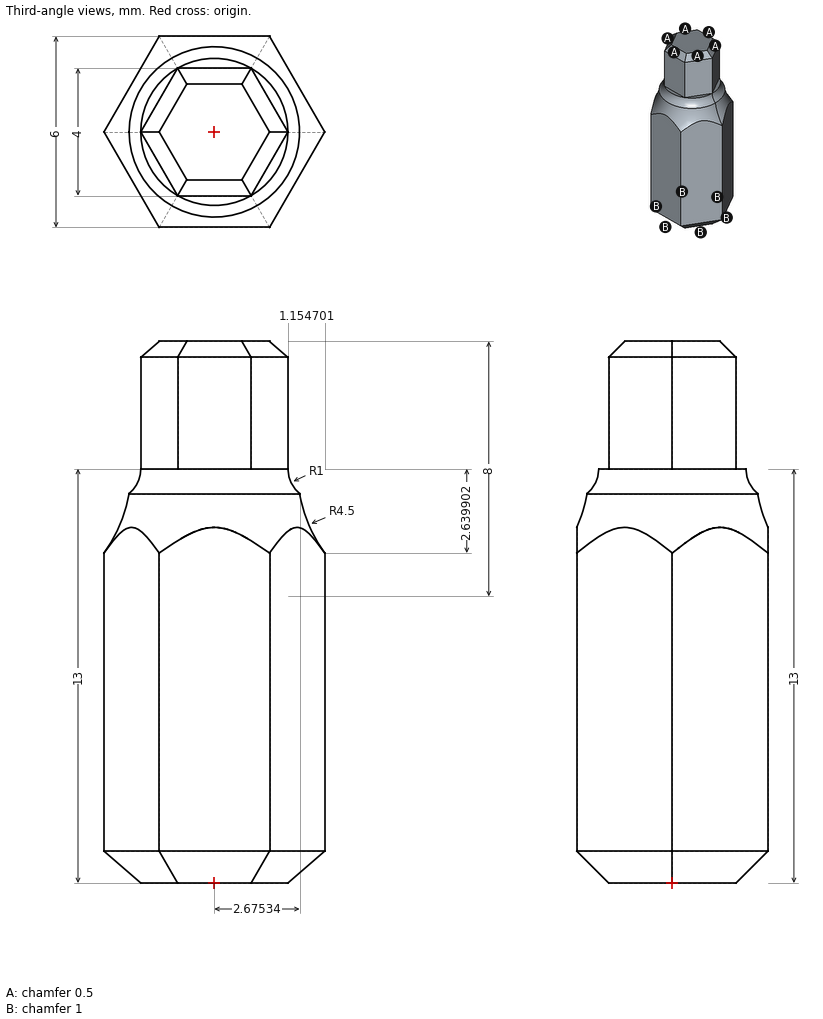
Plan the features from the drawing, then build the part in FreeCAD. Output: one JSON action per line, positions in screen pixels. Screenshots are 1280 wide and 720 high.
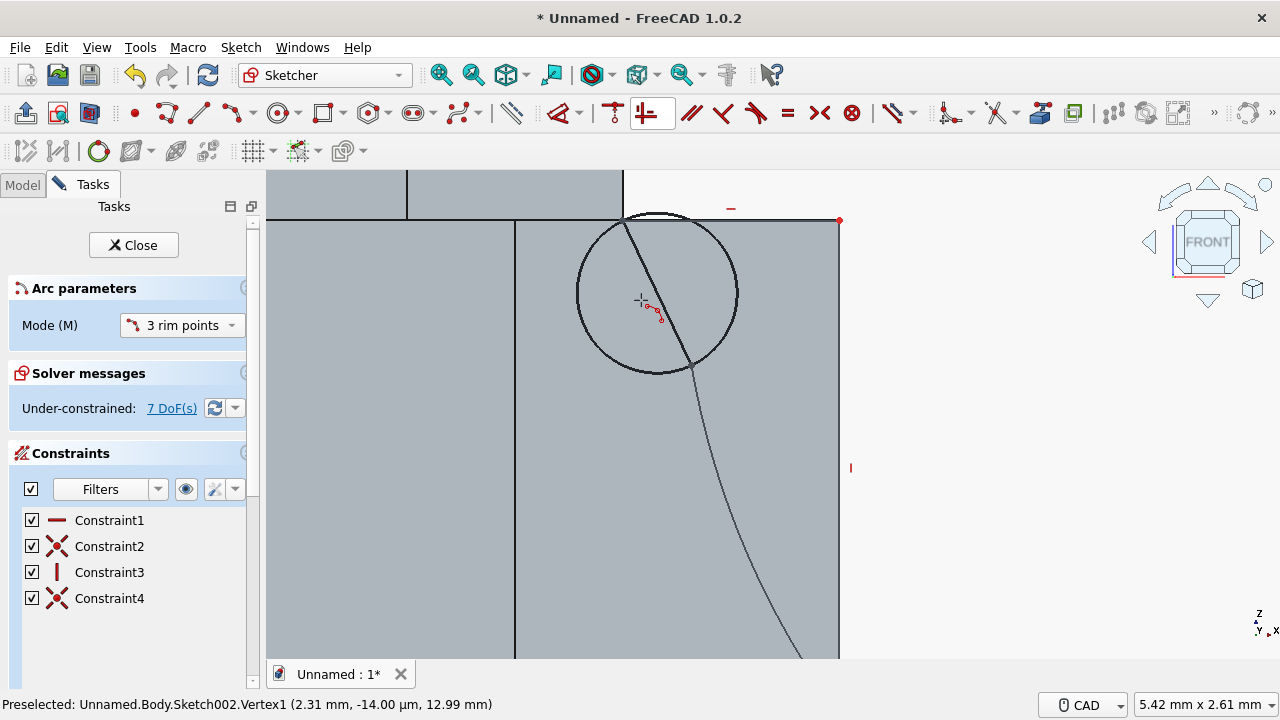
{"action": "left_click", "coordinate": [641, 300]}
{"action": "key", "text": "Escape"}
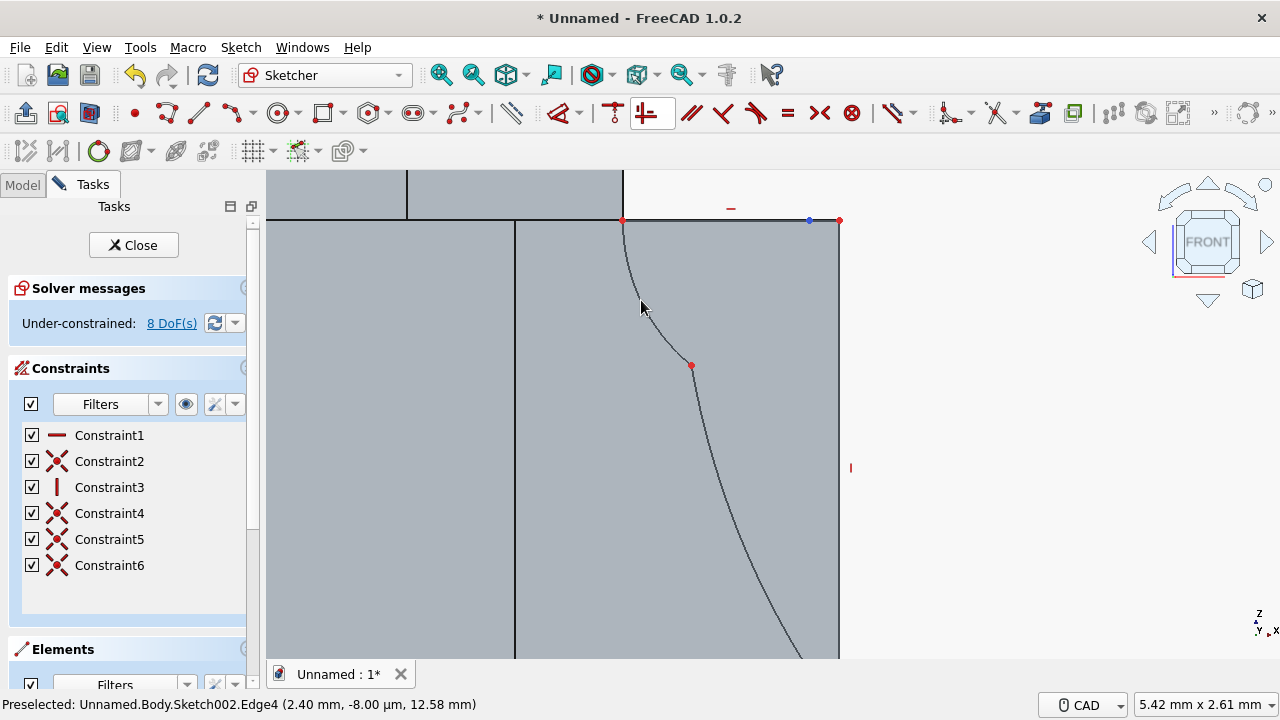
{"action": "left_click", "coordinate": [558, 114]}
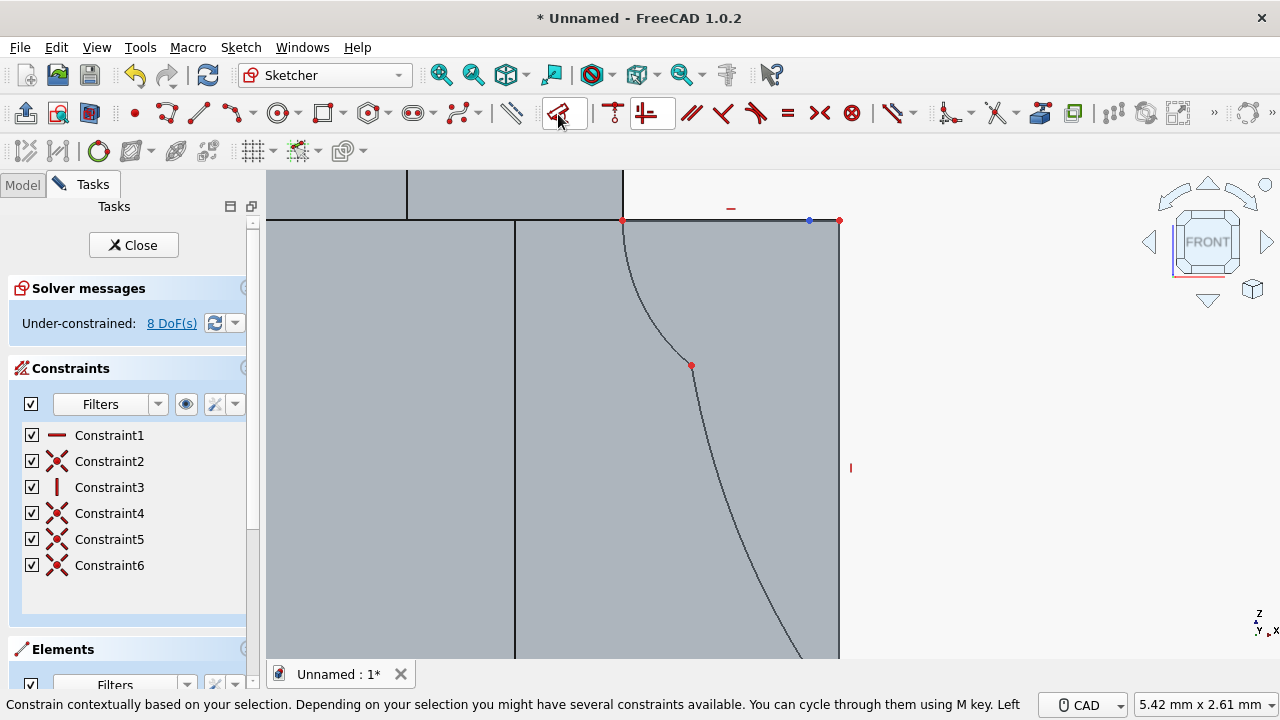
{"action": "left_click", "coordinate": [719, 477]}
{"action": "left_click", "coordinate": [689, 487]}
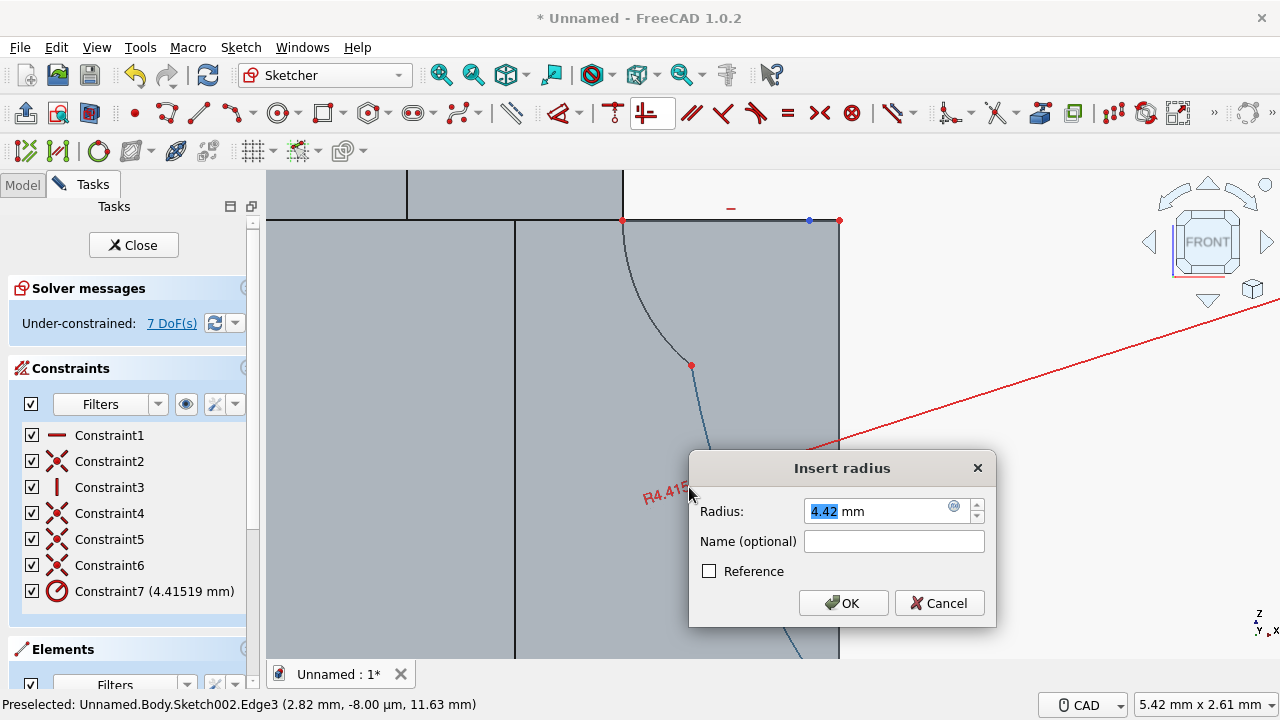
{"action": "type", "text": "4.5"}
{"action": "key", "text": "Return"}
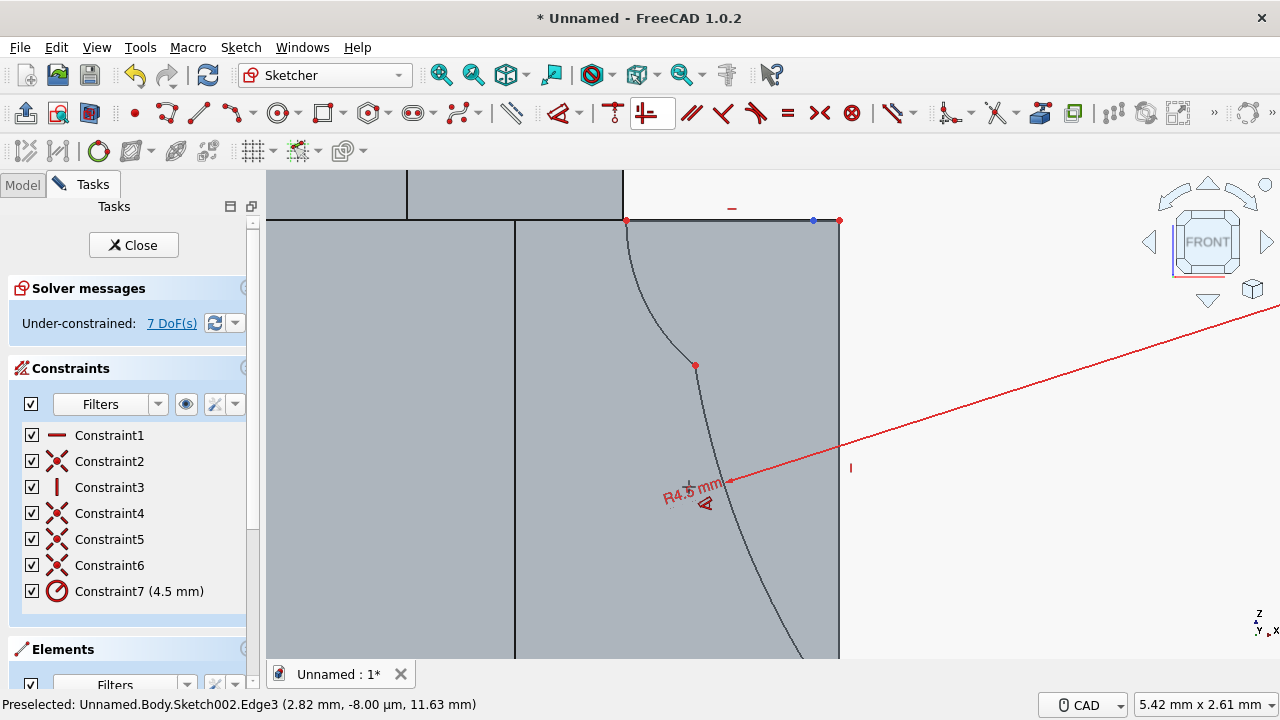
{"action": "left_click", "coordinate": [633, 270]}
{"action": "left_click", "coordinate": [602, 278]}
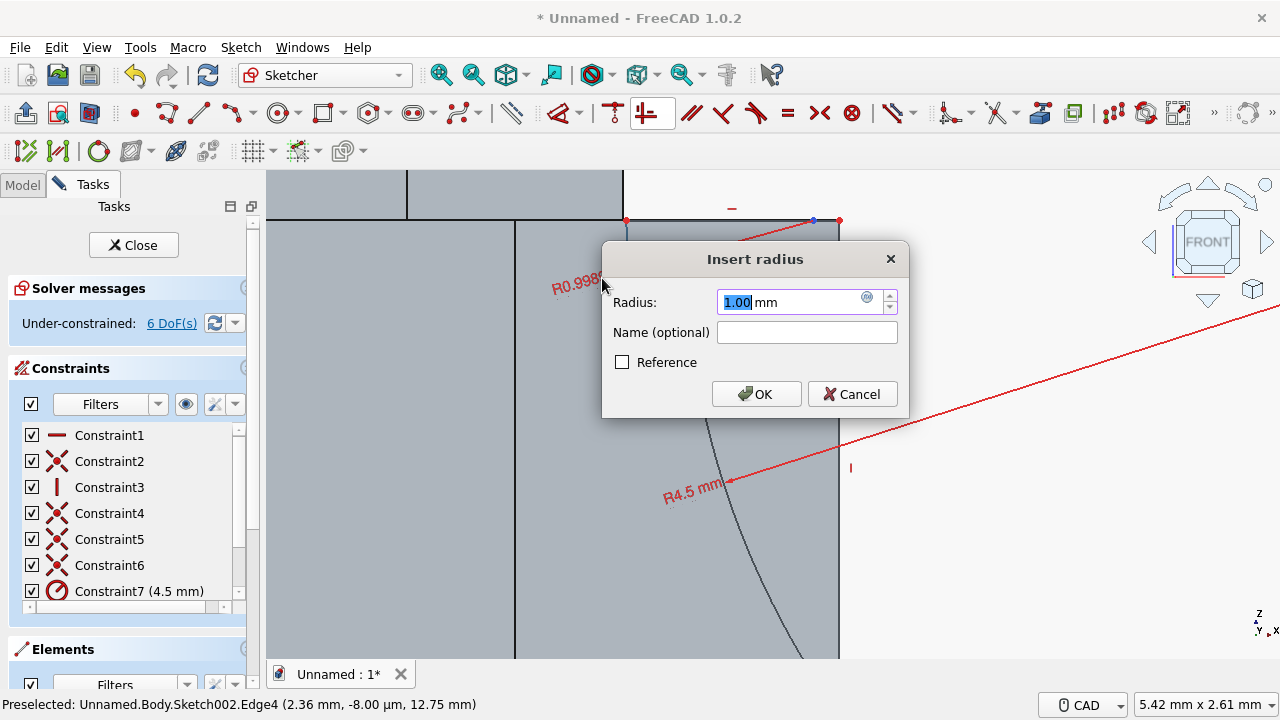
{"action": "type", "text": "1"}
{"action": "key", "text": "Return"}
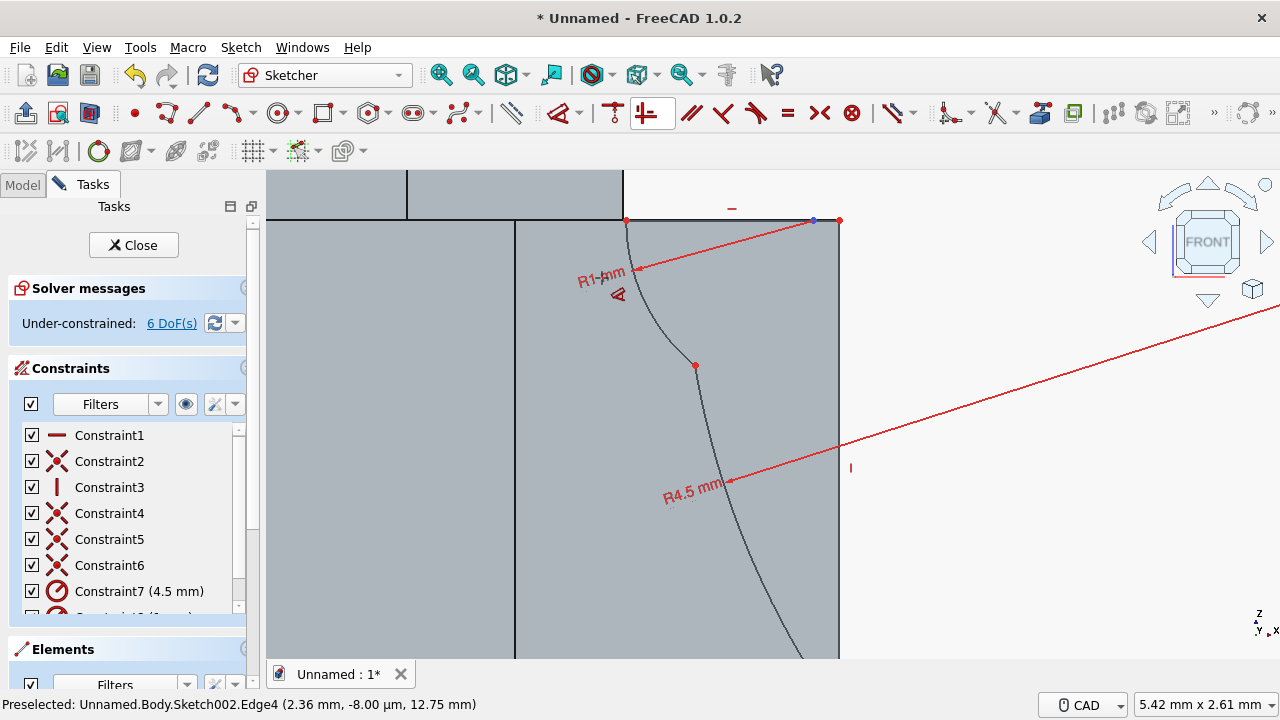
{"action": "left_click", "coordinate": [626, 221]}
{"action": "left_click", "coordinate": [660, 426]}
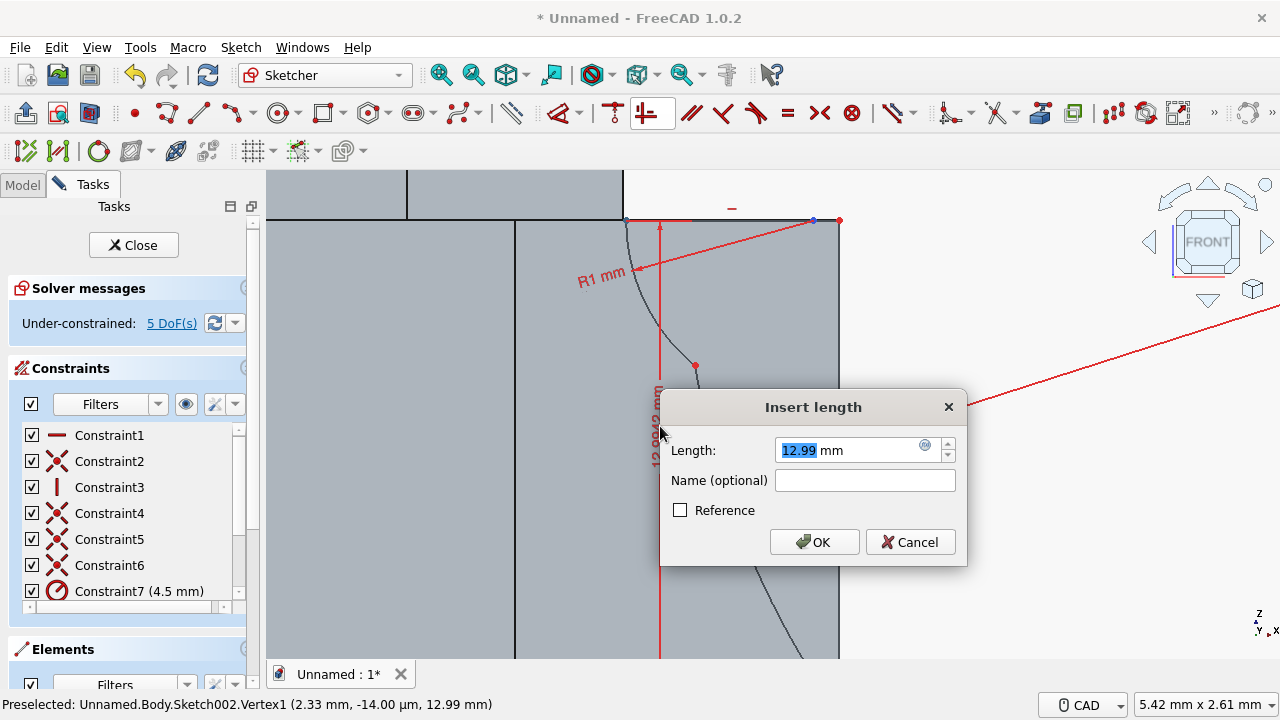
{"action": "type", "text": "13"}
{"action": "key", "text": "Return"}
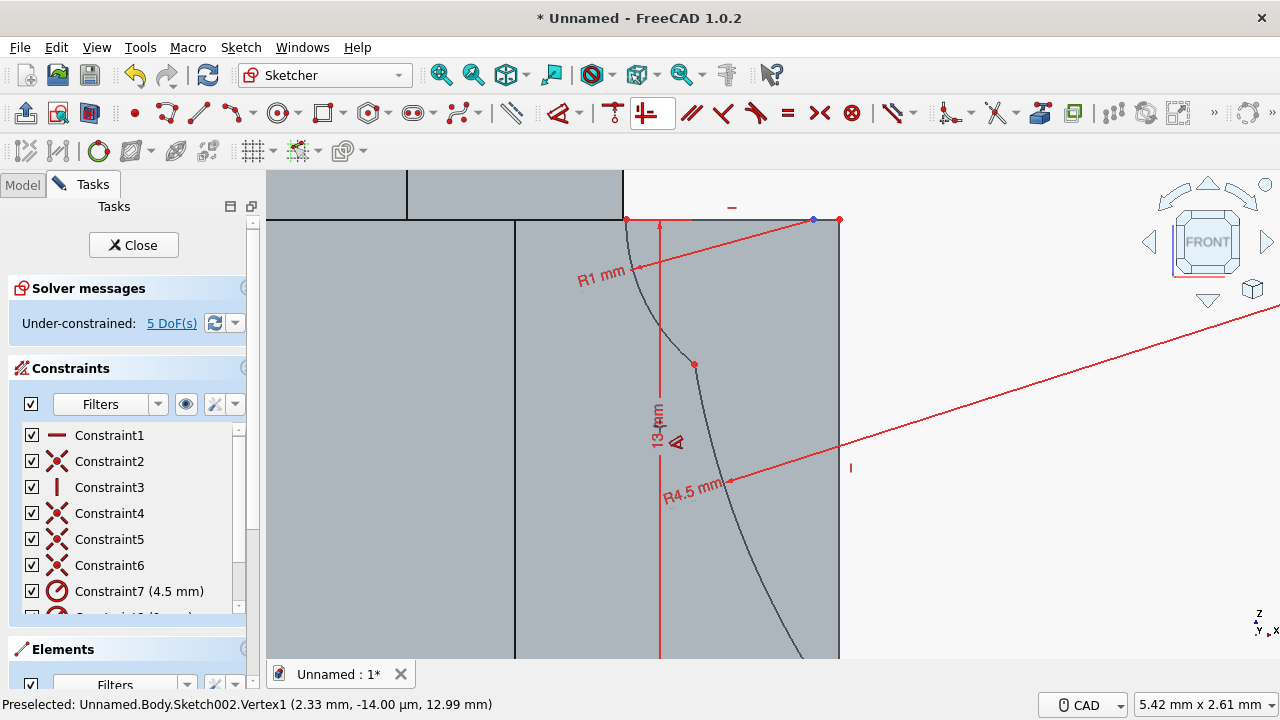
{"action": "scroll", "coordinate": [650, 308], "scroll_direction": "down", "scroll_amount": 2}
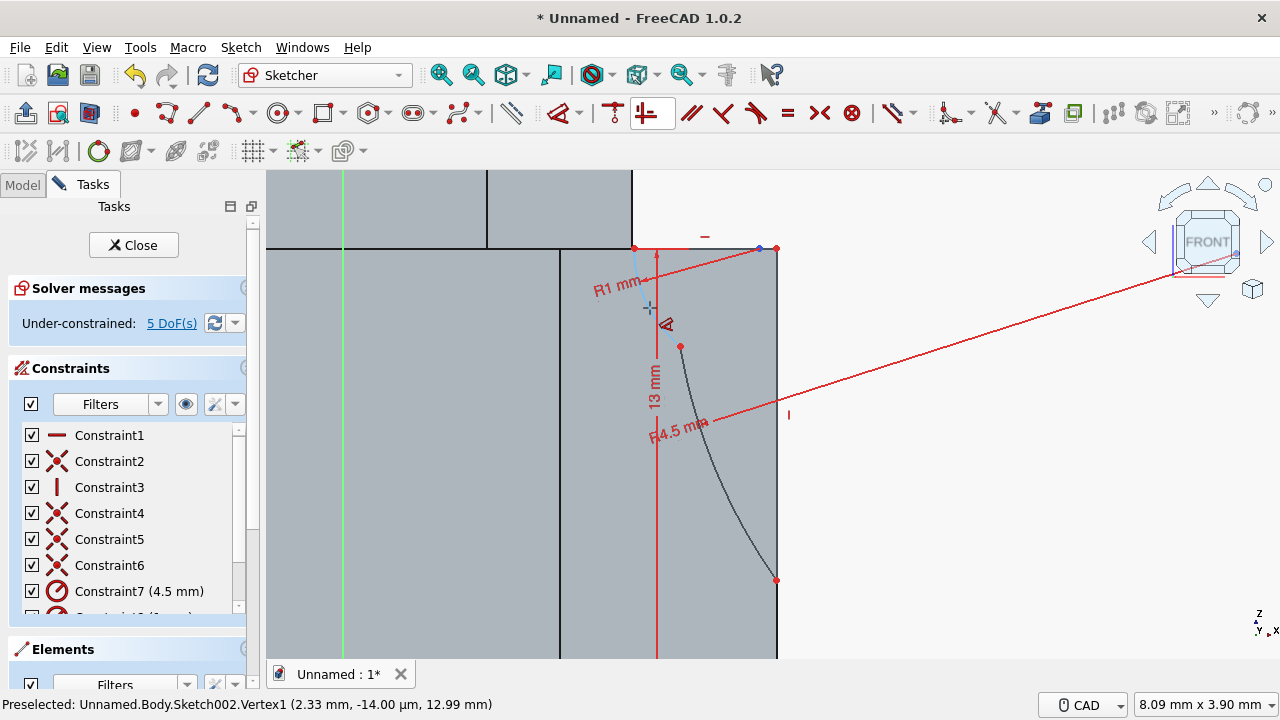
{"action": "scroll", "coordinate": [294, 415], "scroll_direction": "down", "scroll_amount": 1}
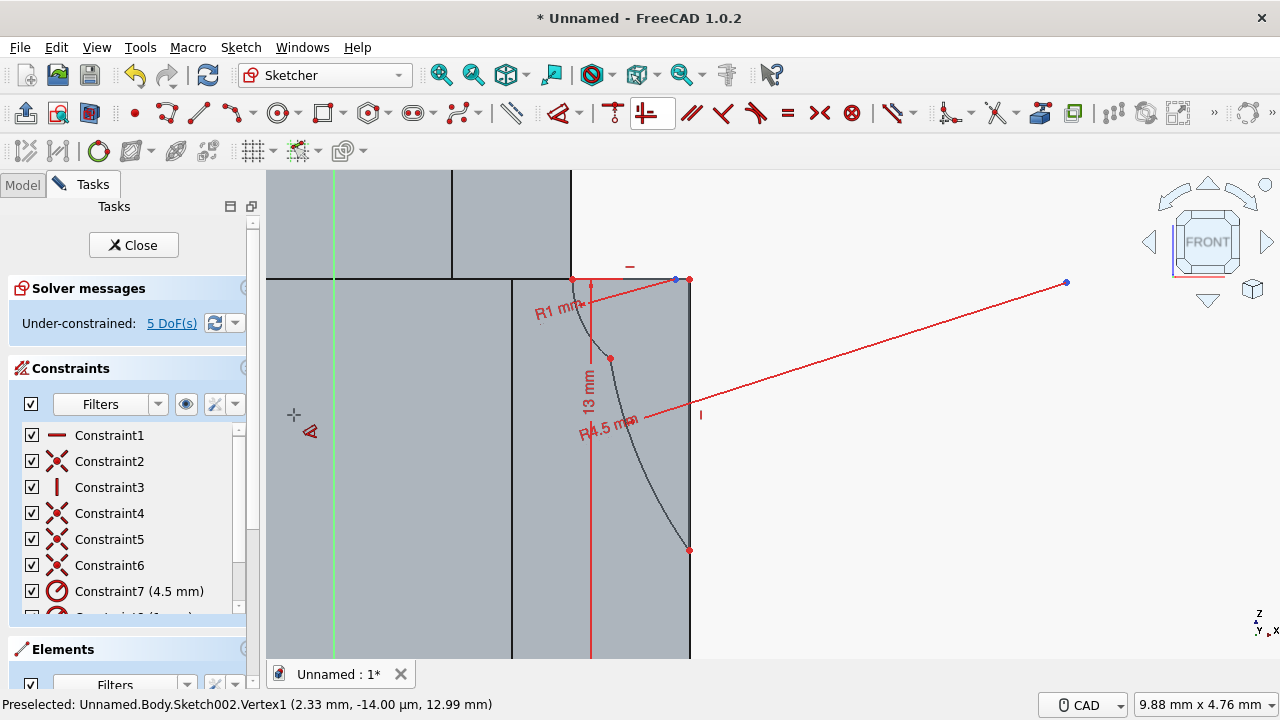
{"action": "left_click", "coordinate": [1066, 283]}
{"action": "left_click", "coordinate": [1100, 457]}